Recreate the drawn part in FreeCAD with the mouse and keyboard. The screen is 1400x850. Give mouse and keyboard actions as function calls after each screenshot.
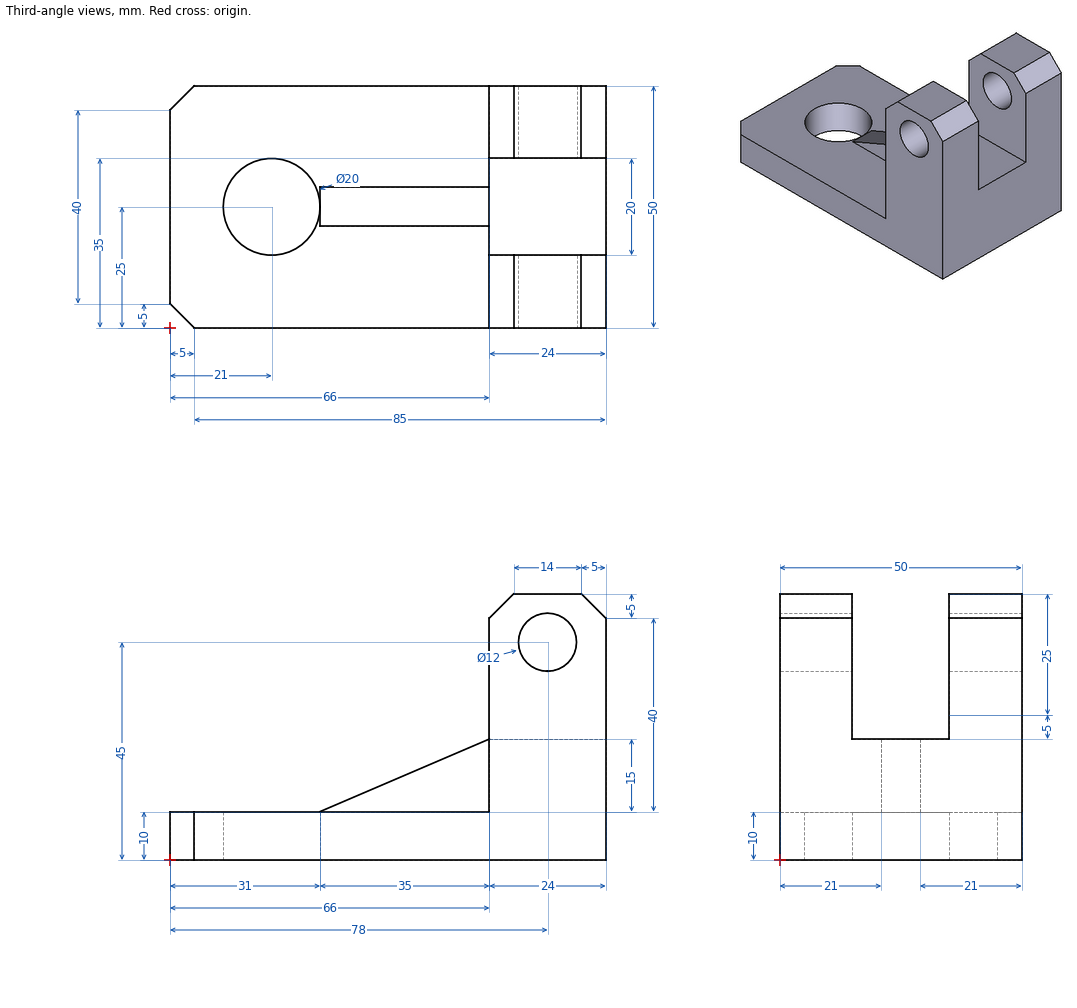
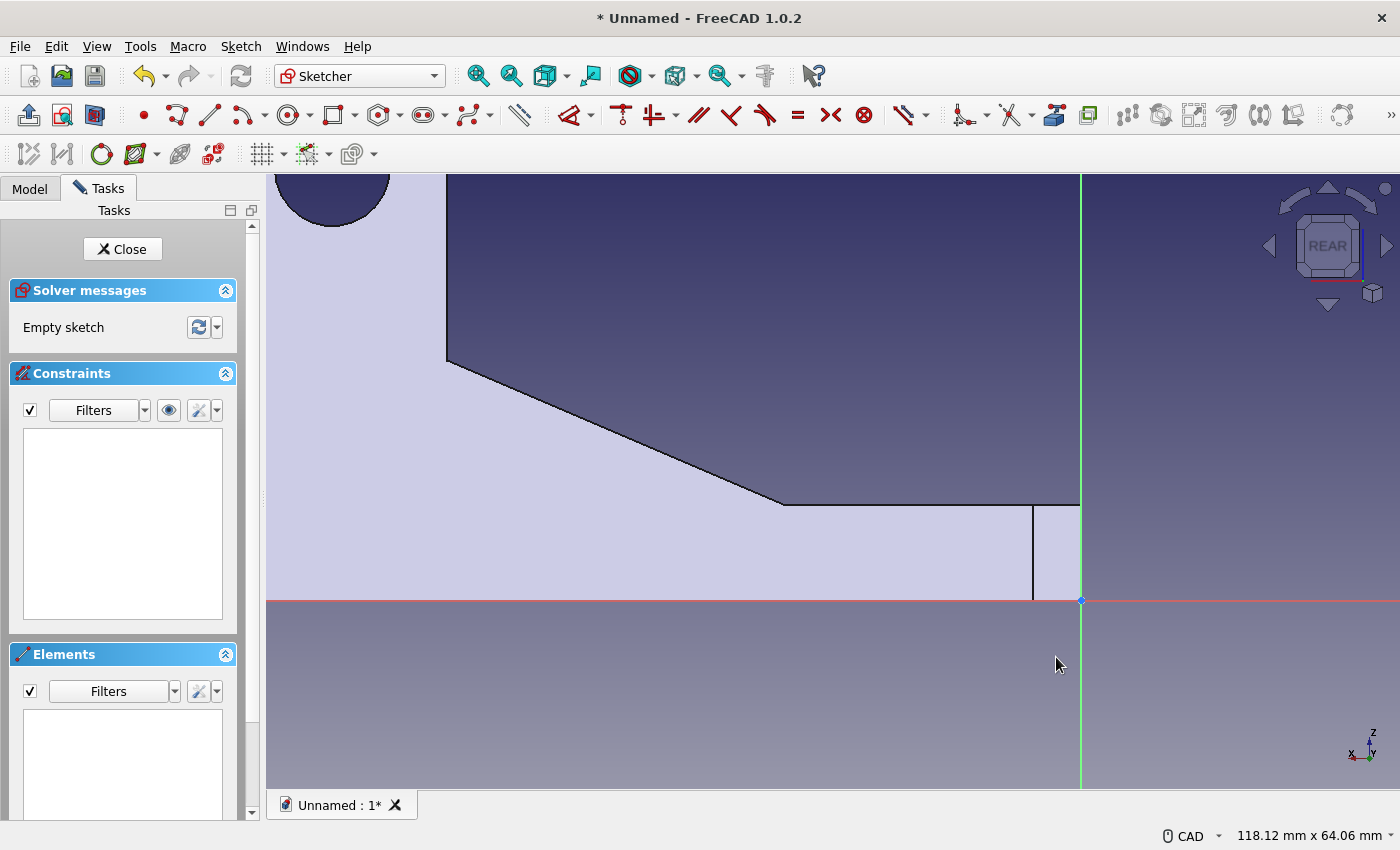
click(177, 116)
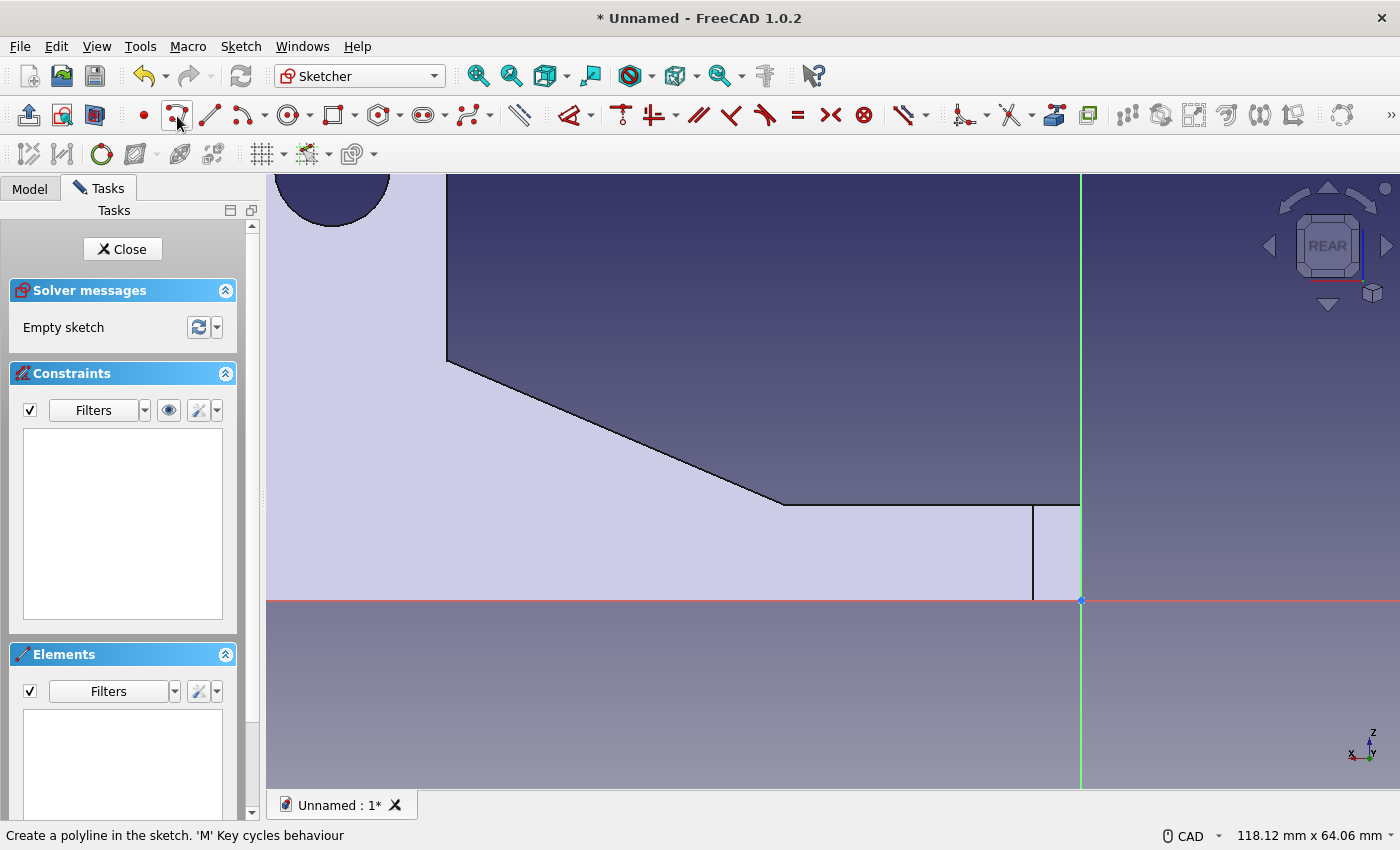
click(783, 505)
click(447, 361)
click(447, 505)
click(783, 506)
key(Escape)
key(Escape)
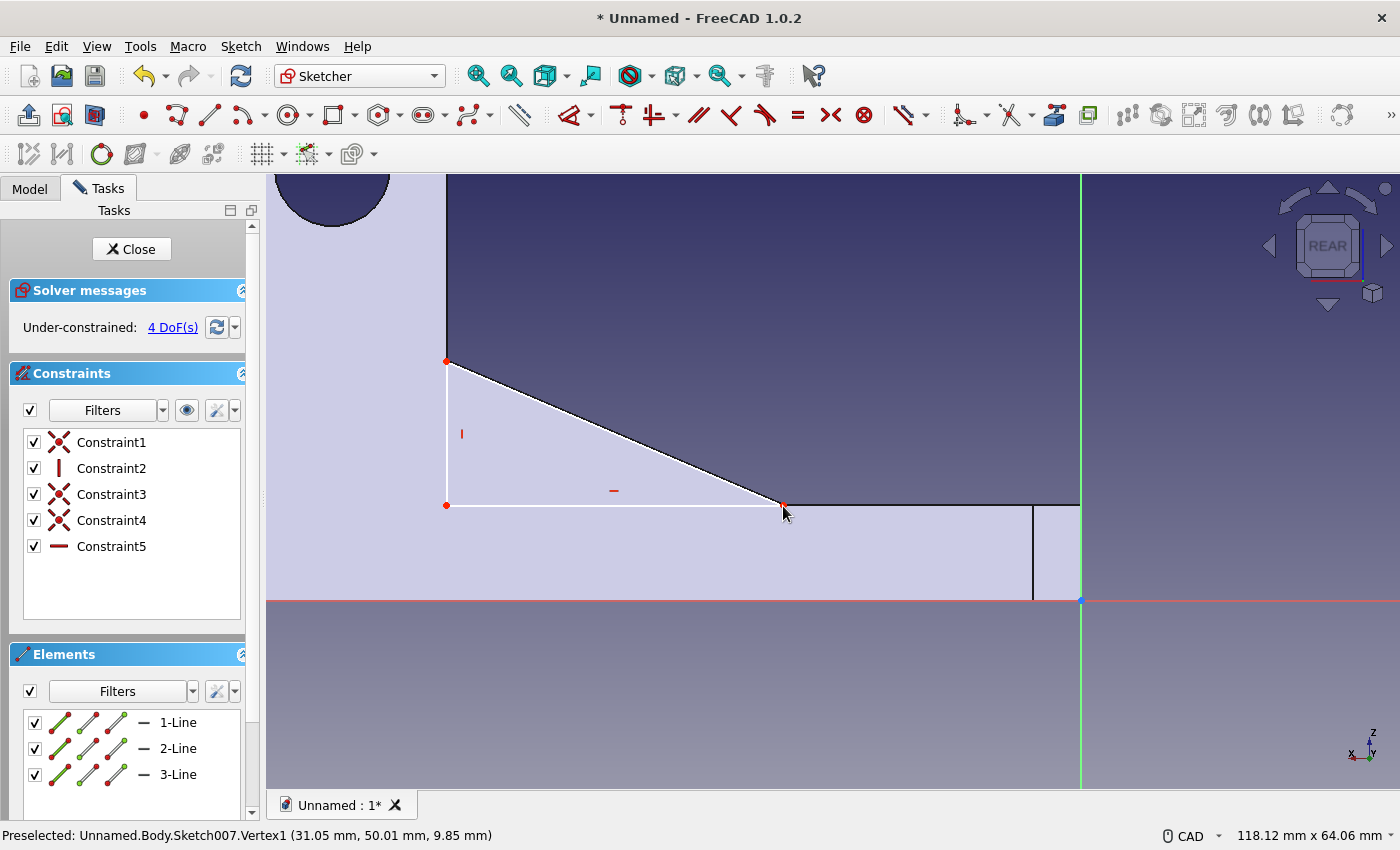
click(568, 116)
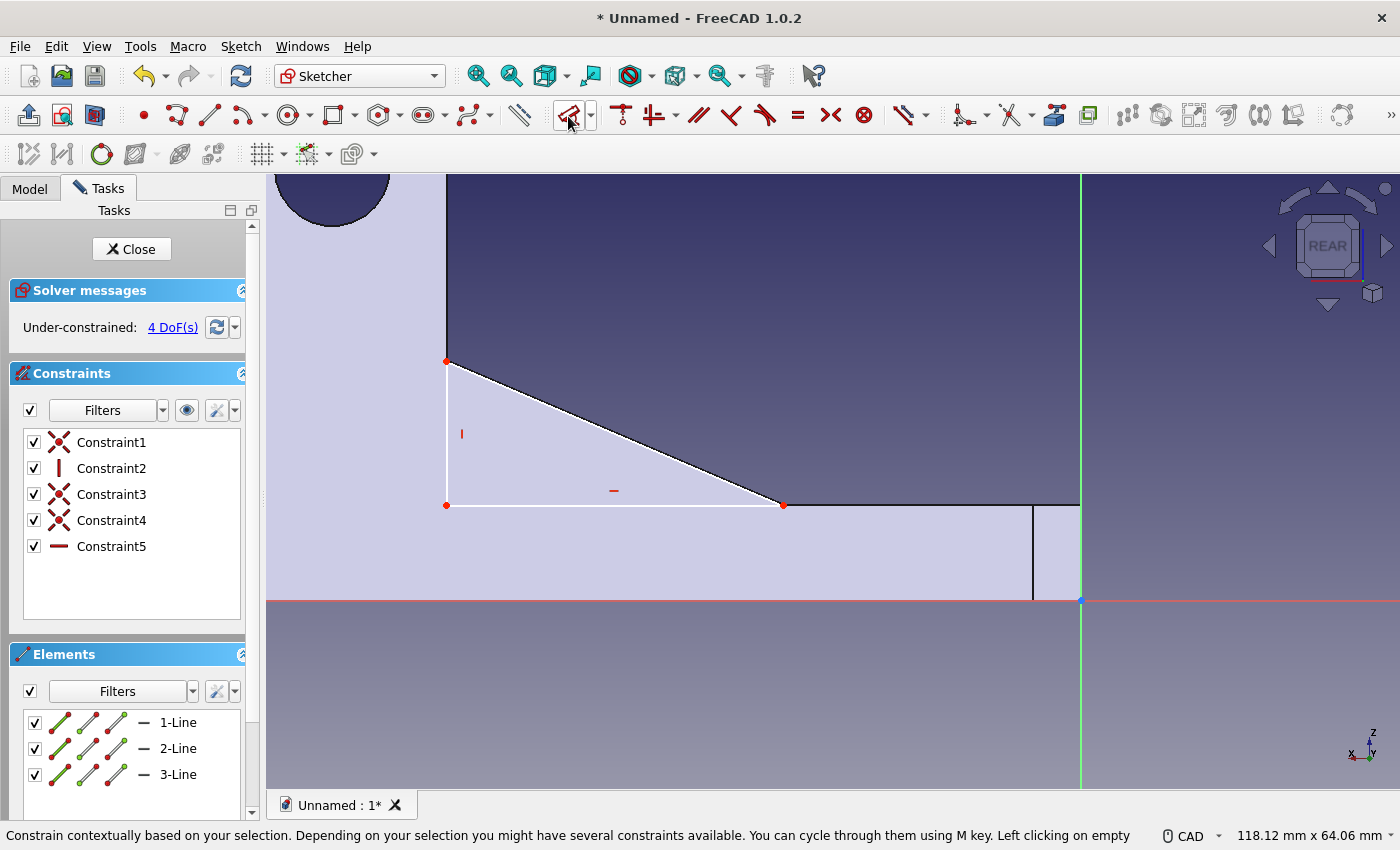
click(447, 405)
click(413, 434)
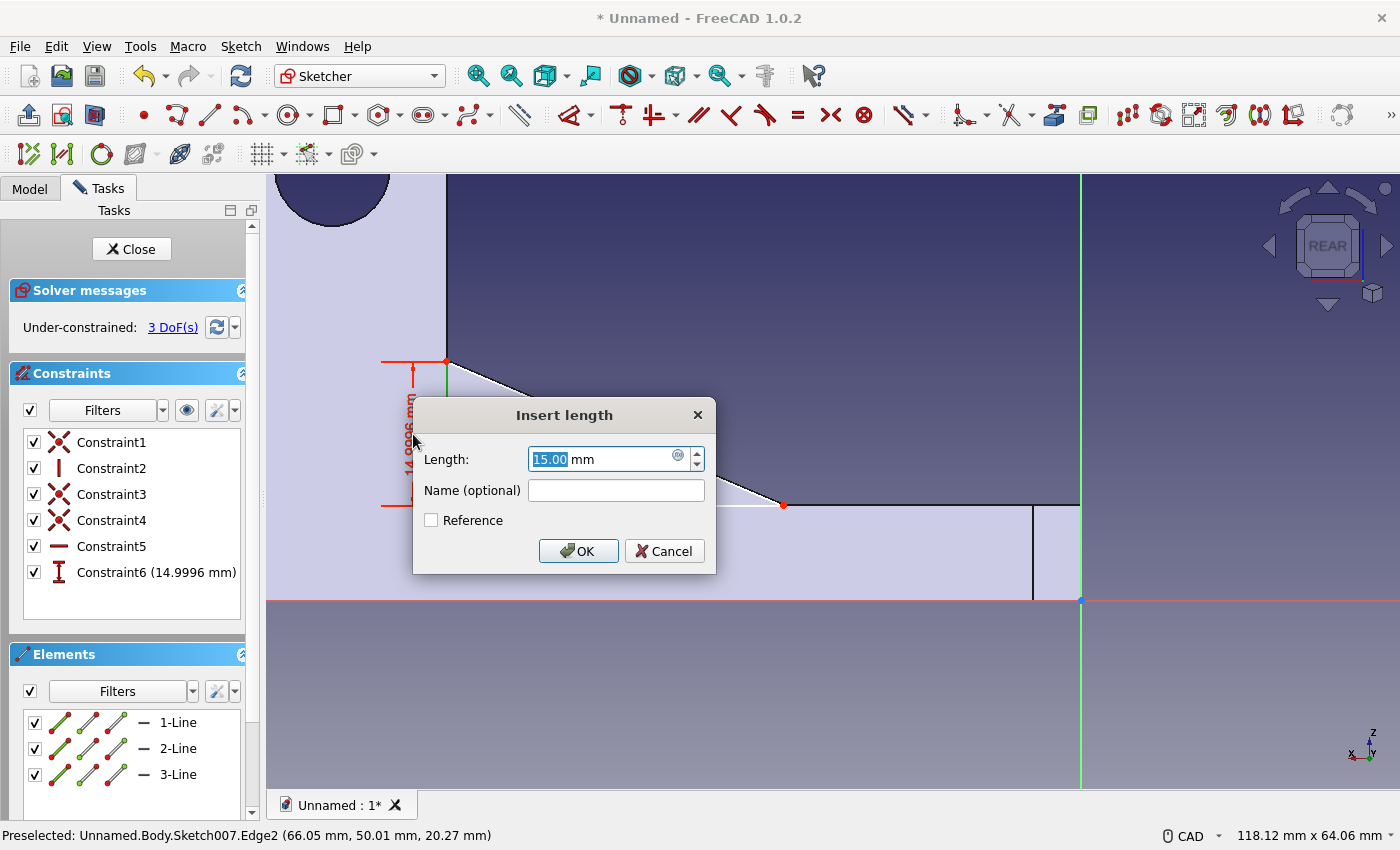
text(15)
key(Return)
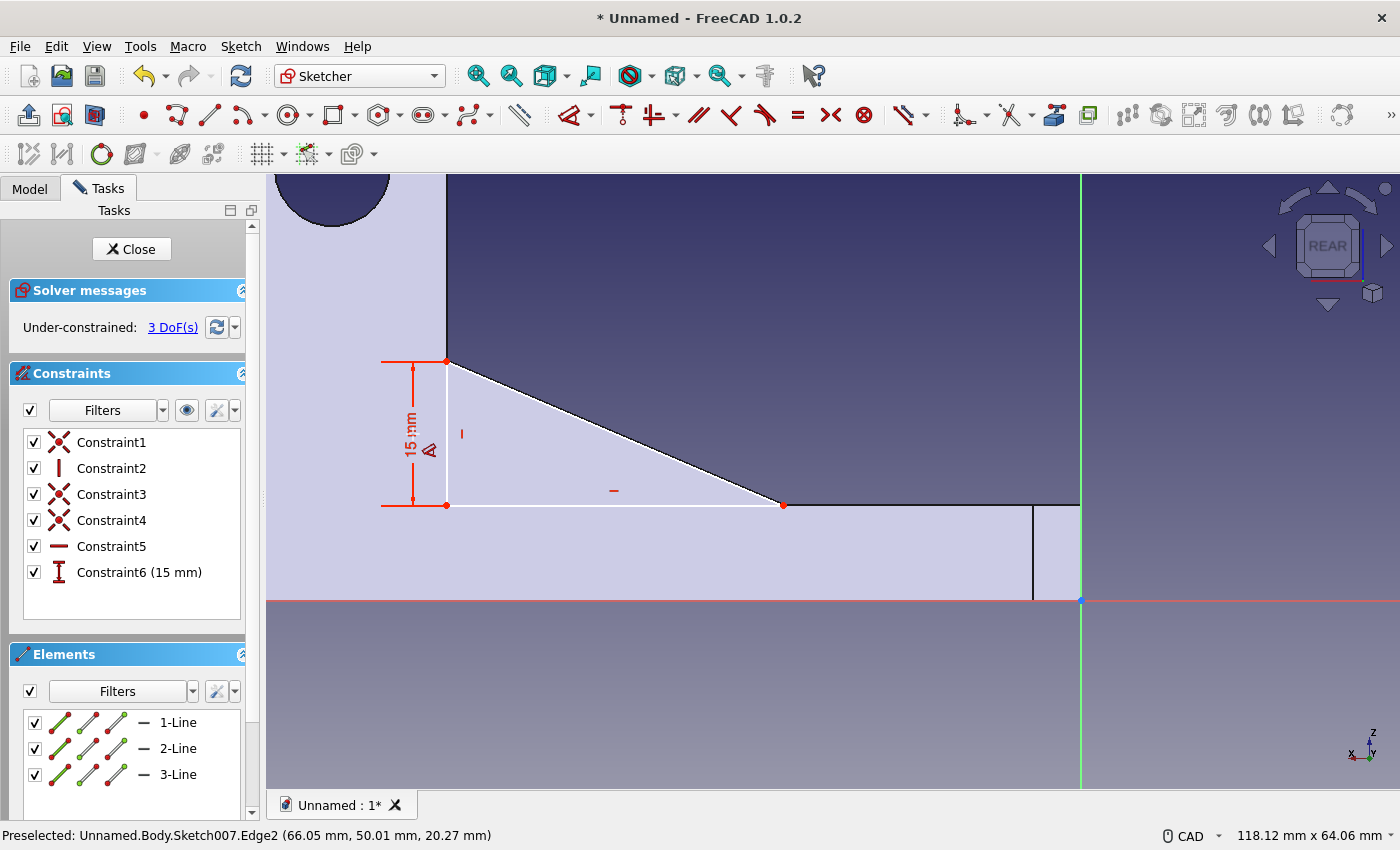
click(548, 506)
click(615, 540)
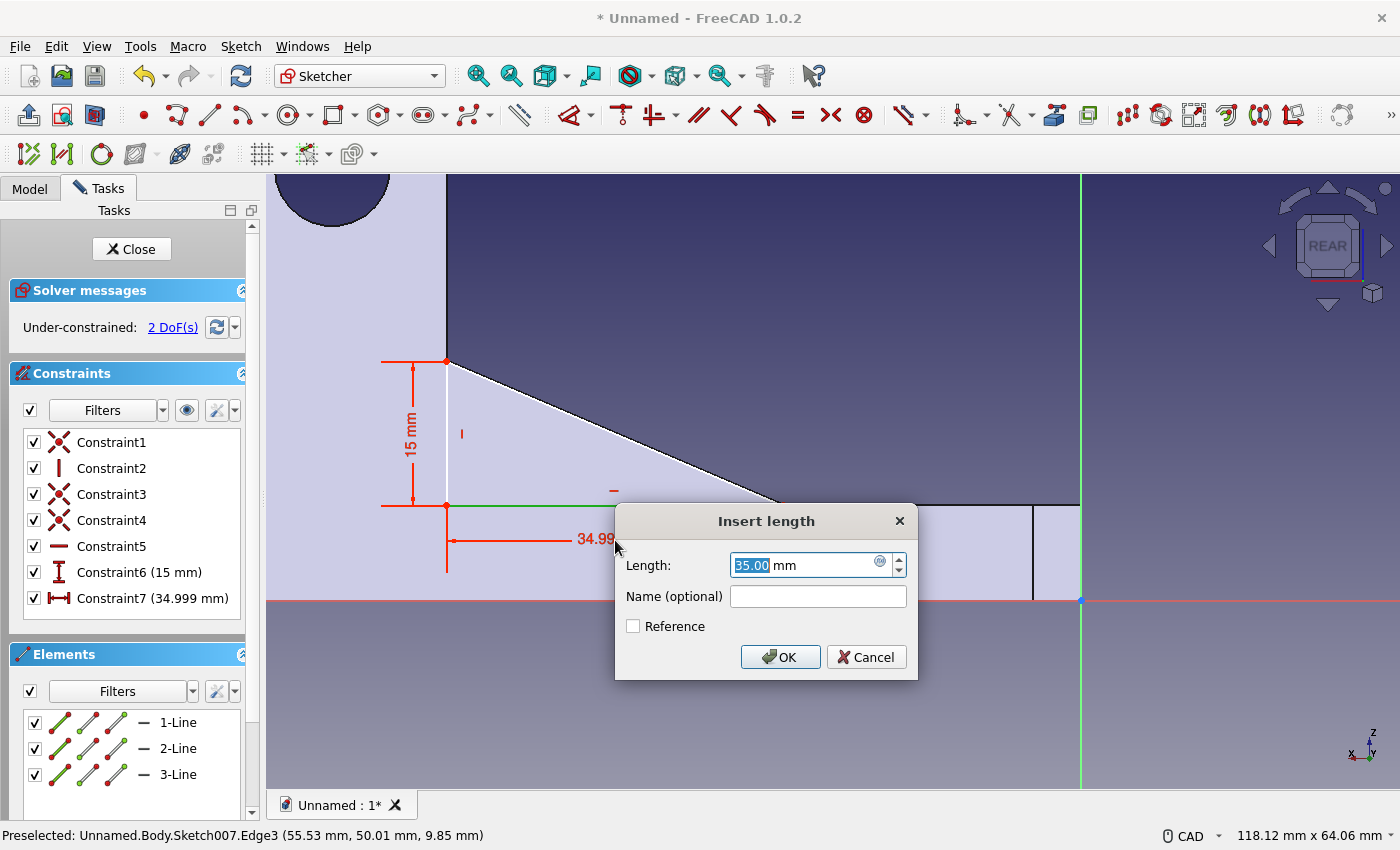
text(35)
key(Return)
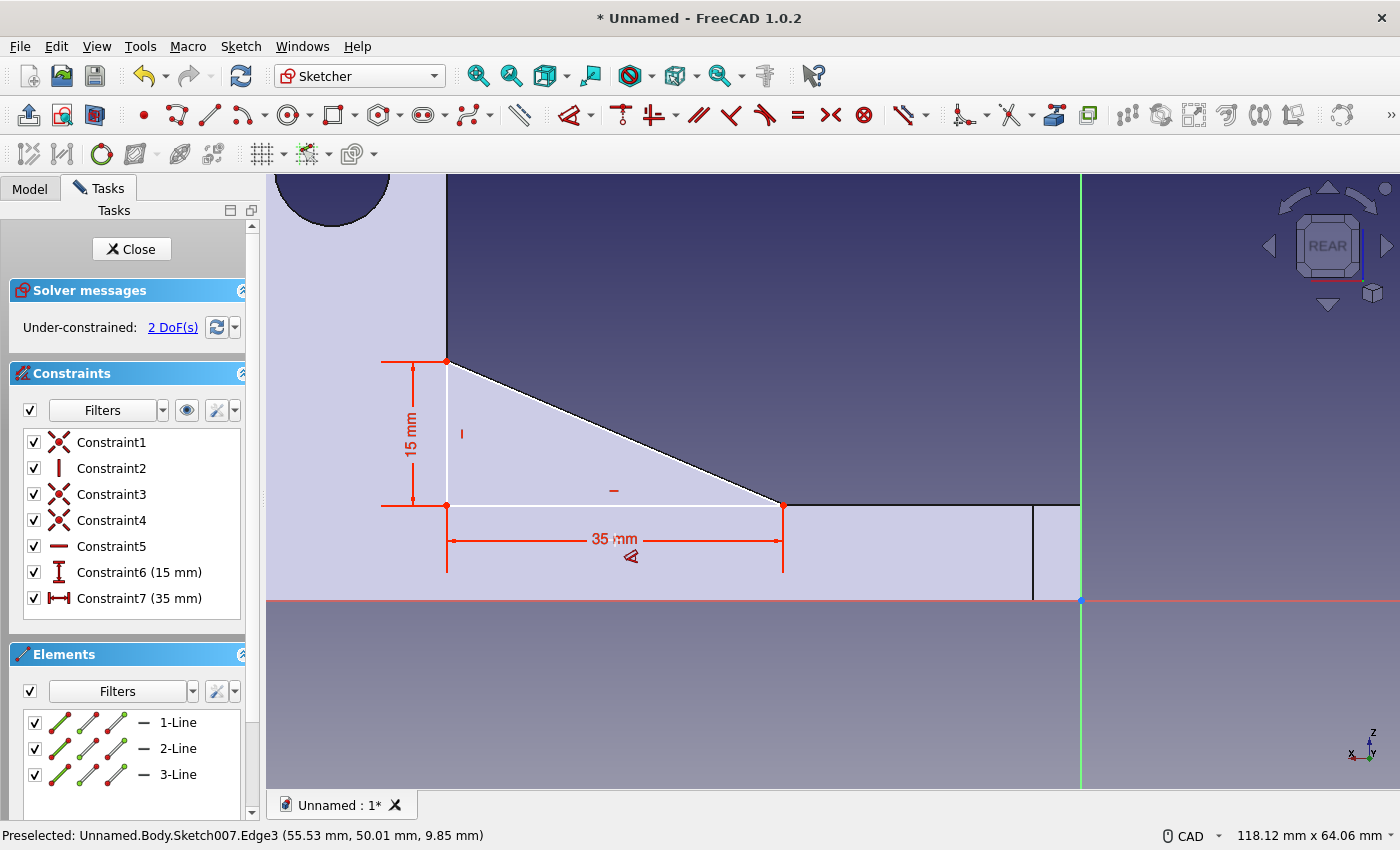
click(783, 506)
click(932, 635)